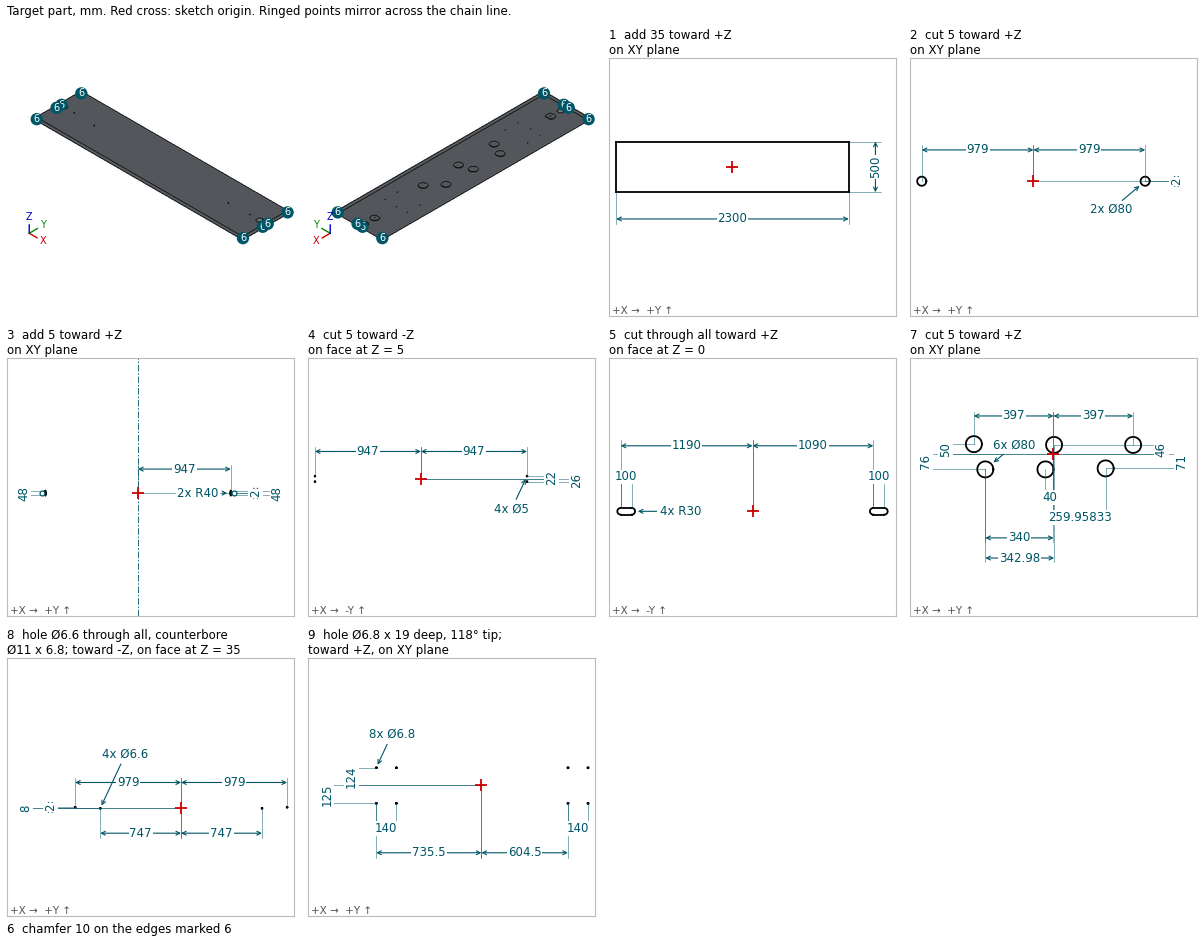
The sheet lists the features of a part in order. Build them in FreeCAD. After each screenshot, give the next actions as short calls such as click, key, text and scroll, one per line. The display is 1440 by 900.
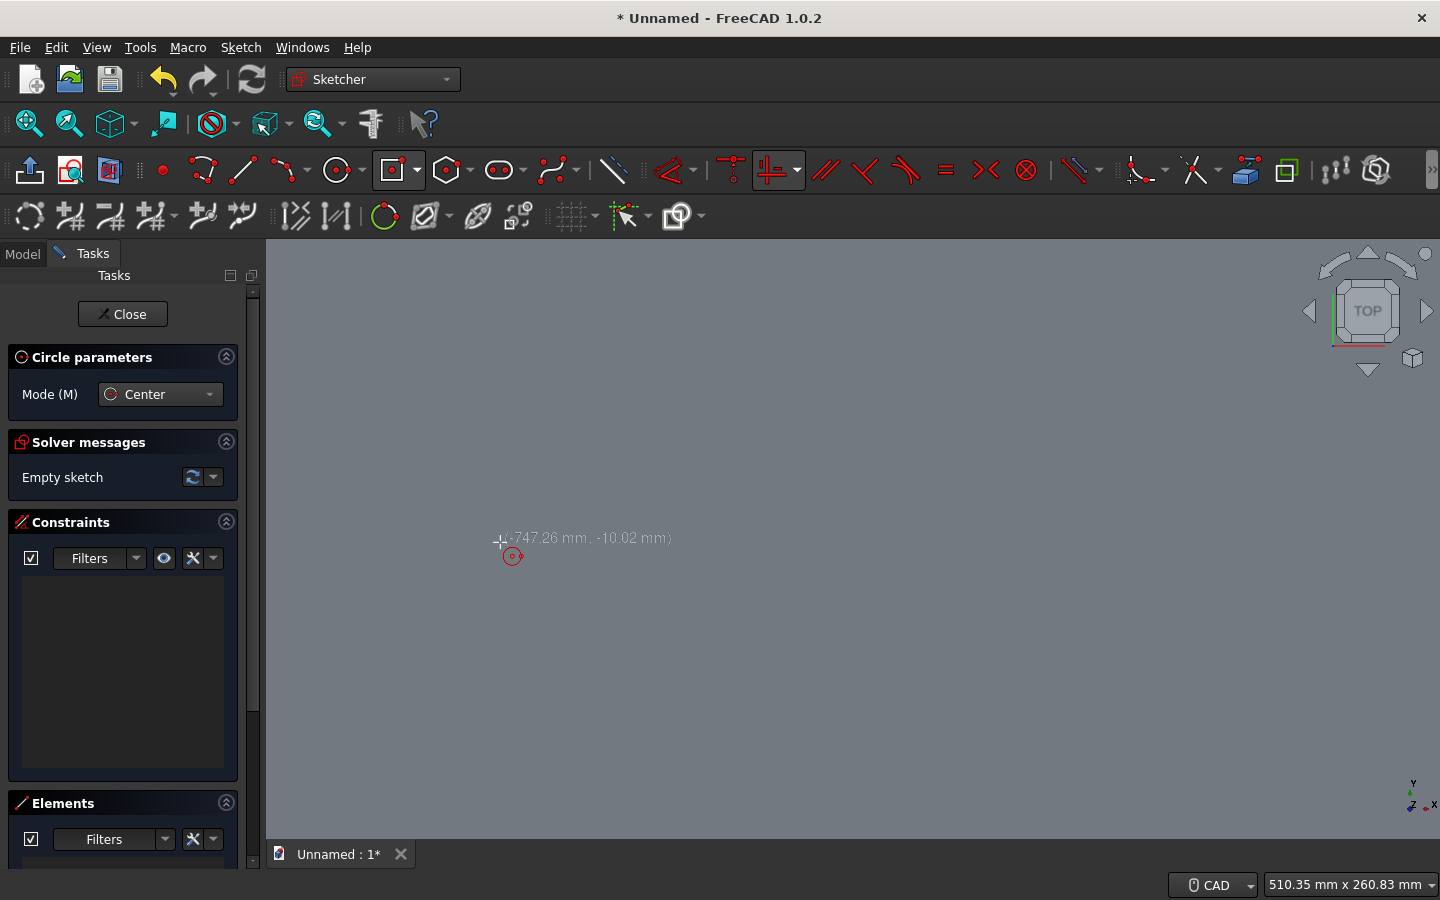
click(501, 538)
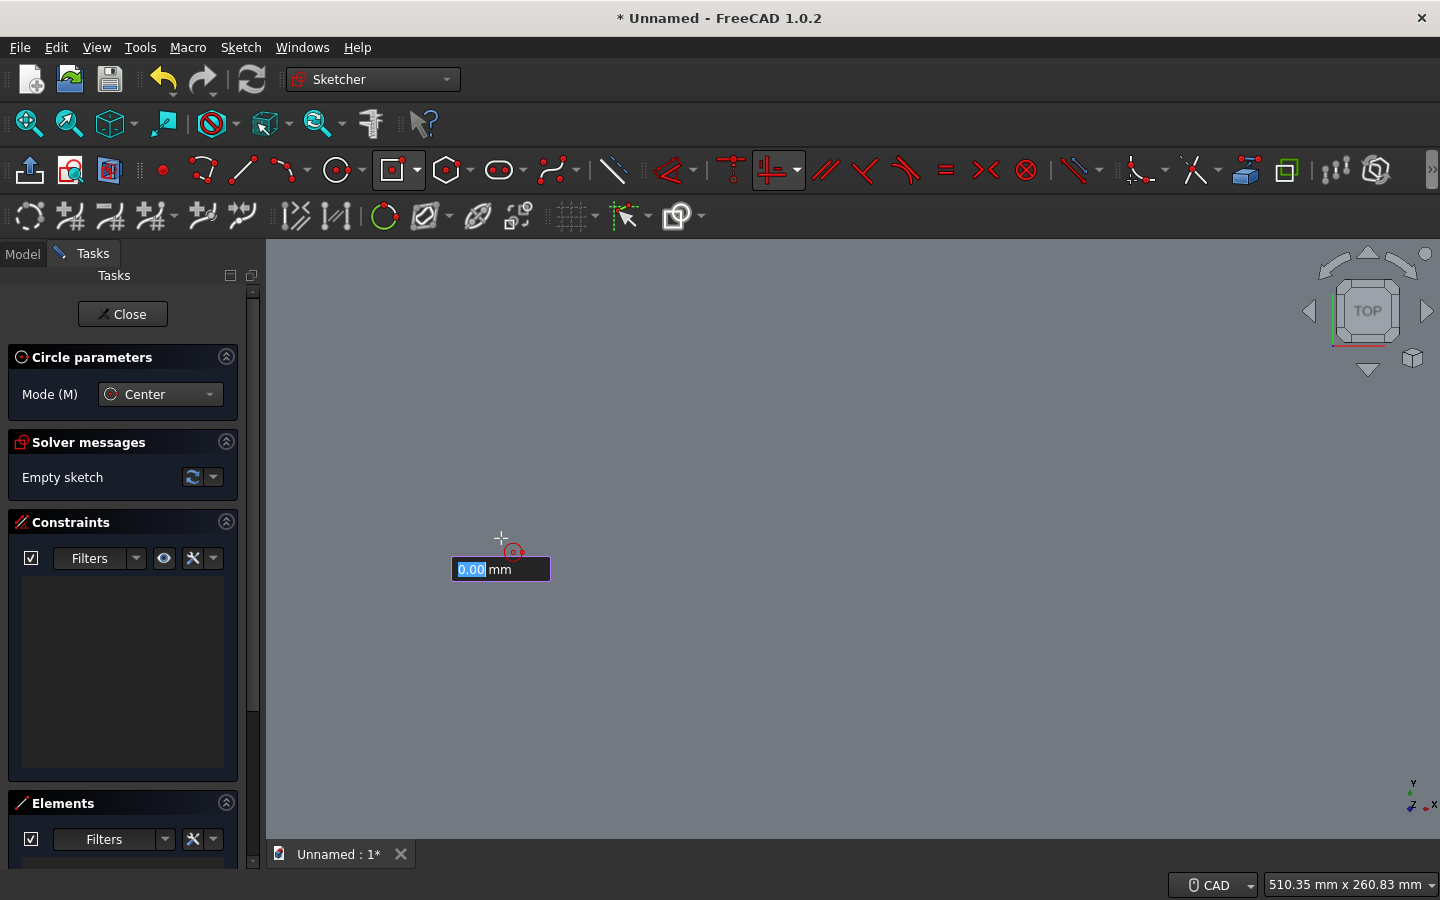
scroll(506, 543, up, 4)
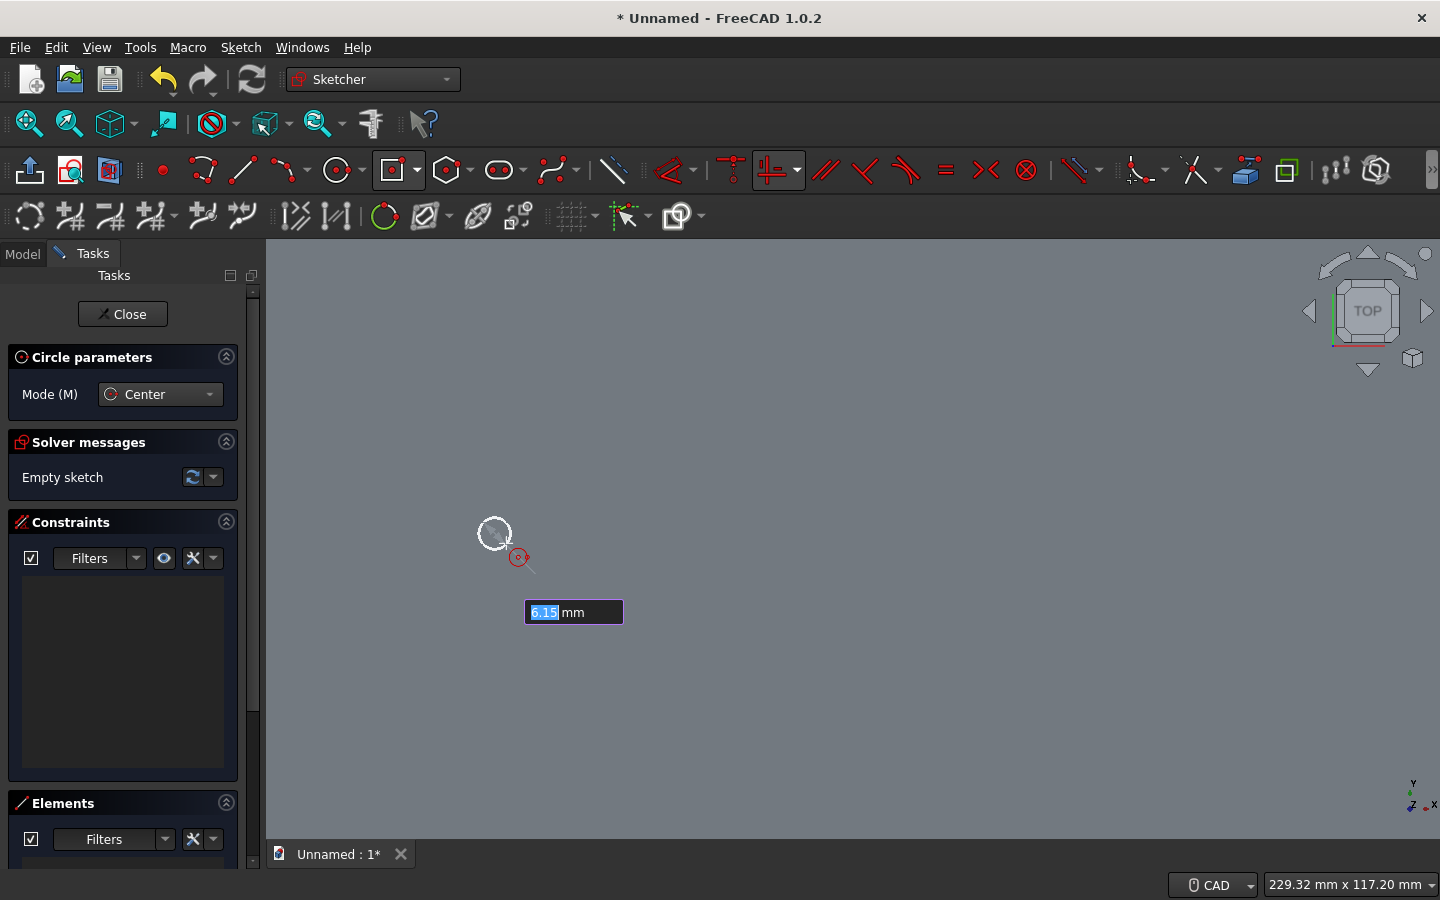
click(506, 543)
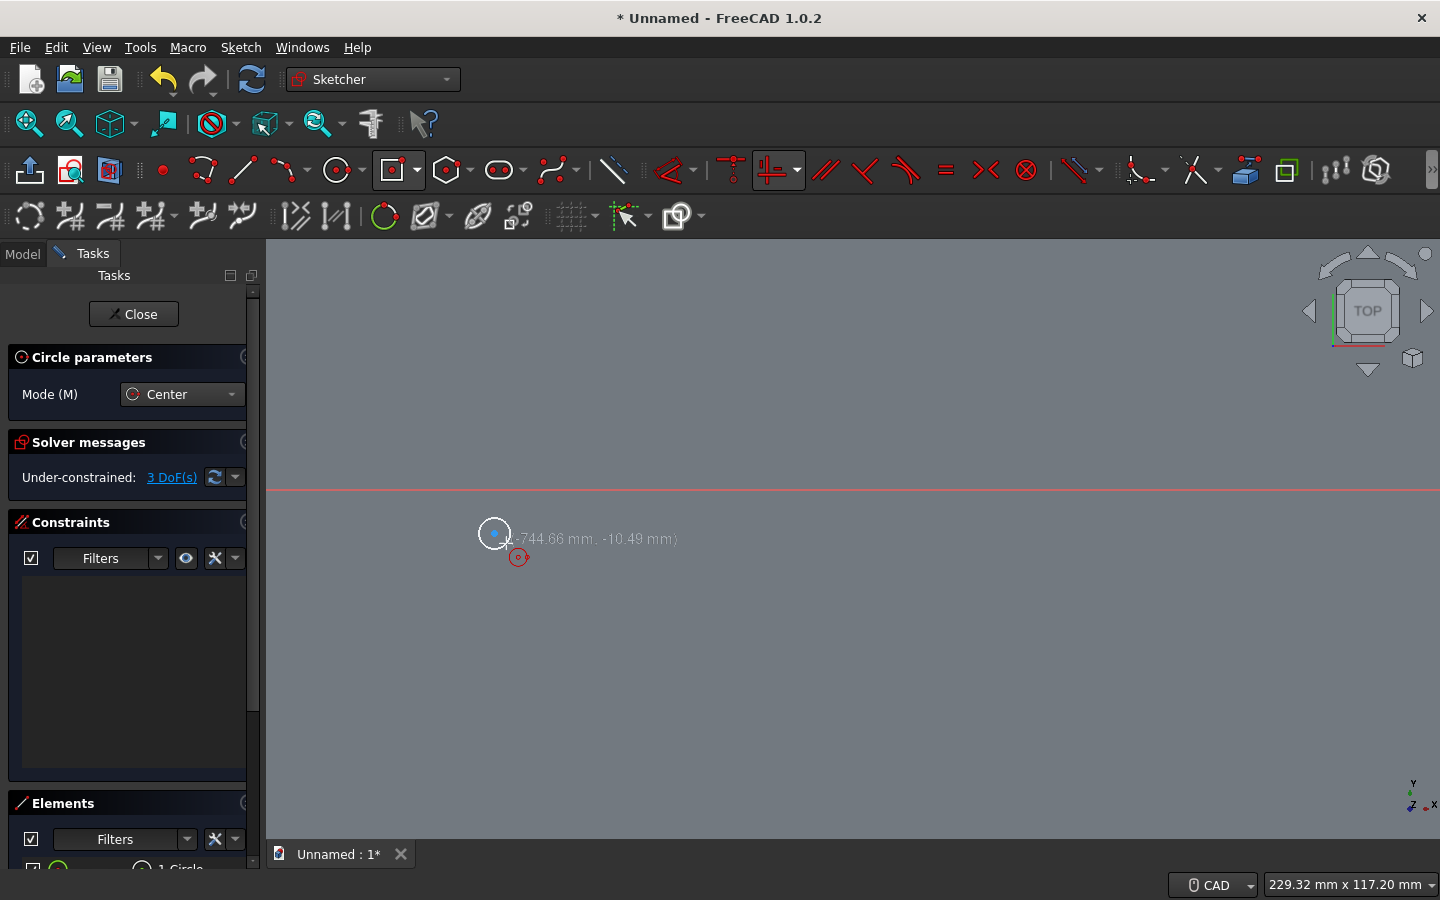
scroll(501, 542, down, 13)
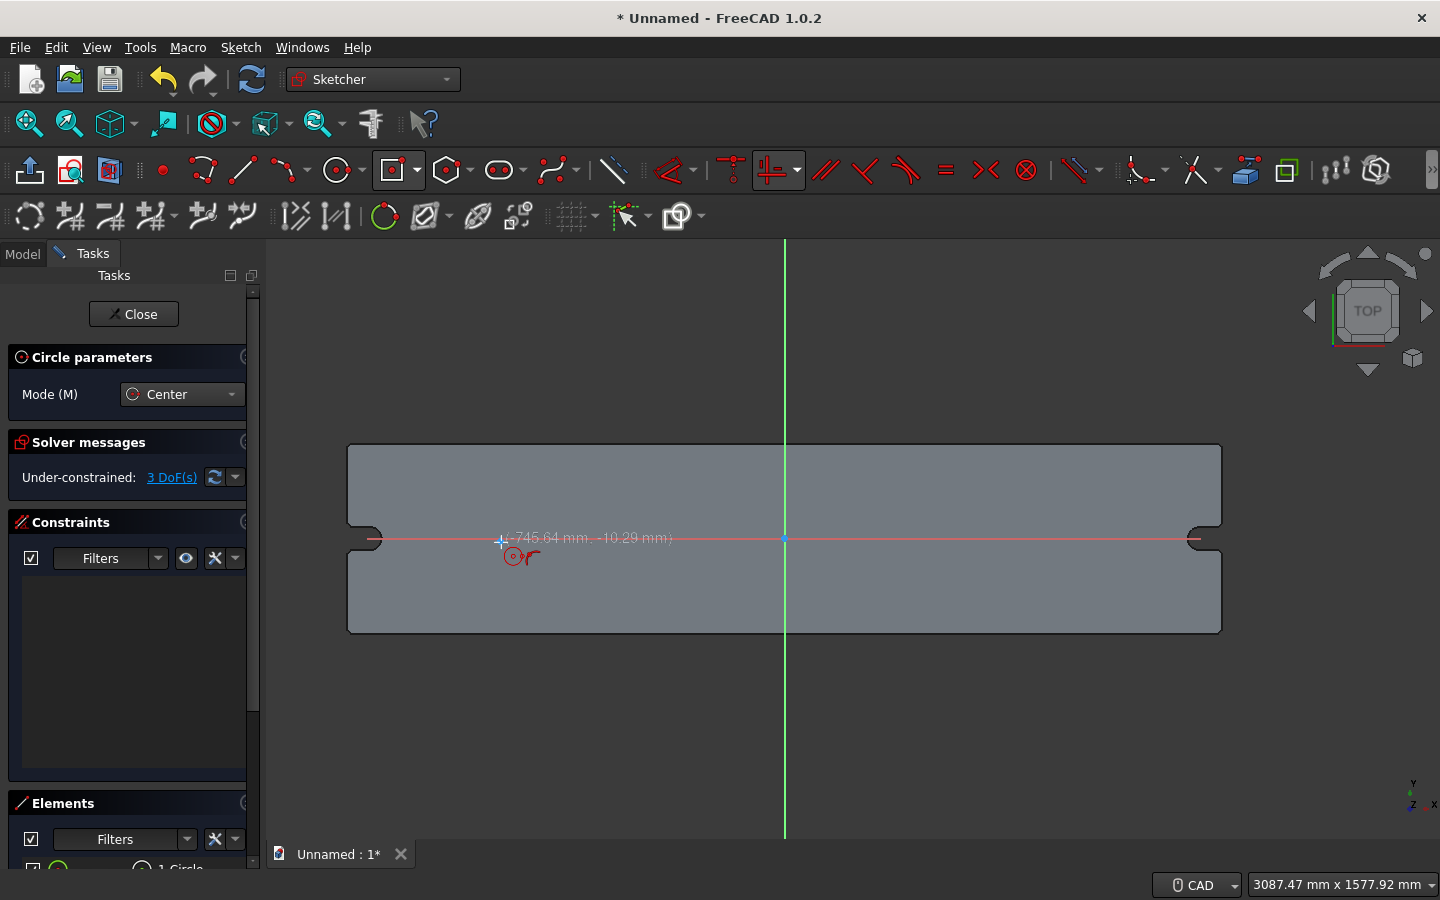
scroll(1069, 542, up, 15)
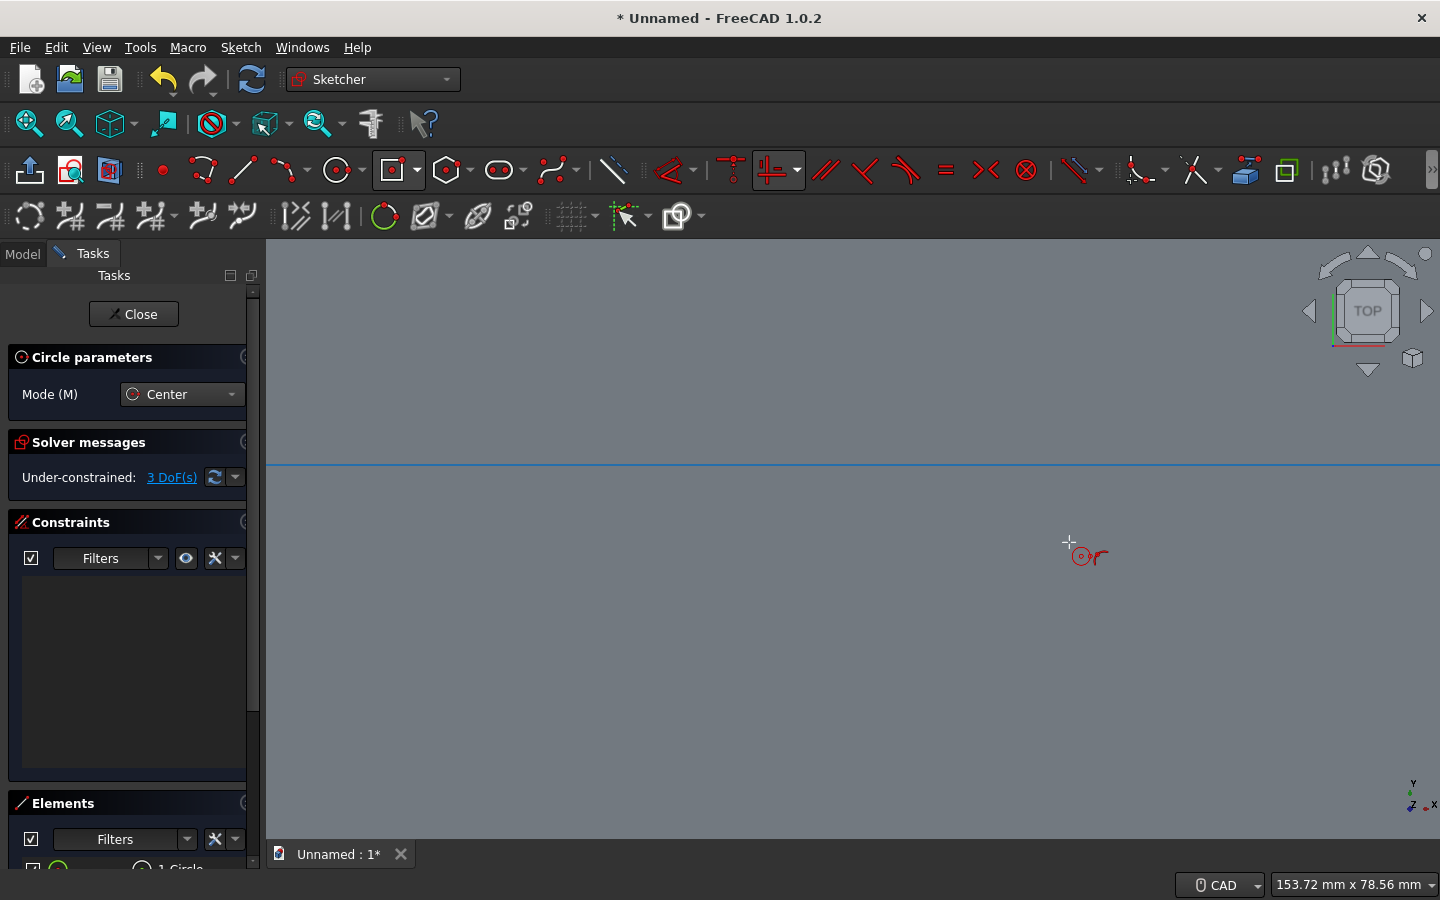
scroll(1069, 542, down, 15)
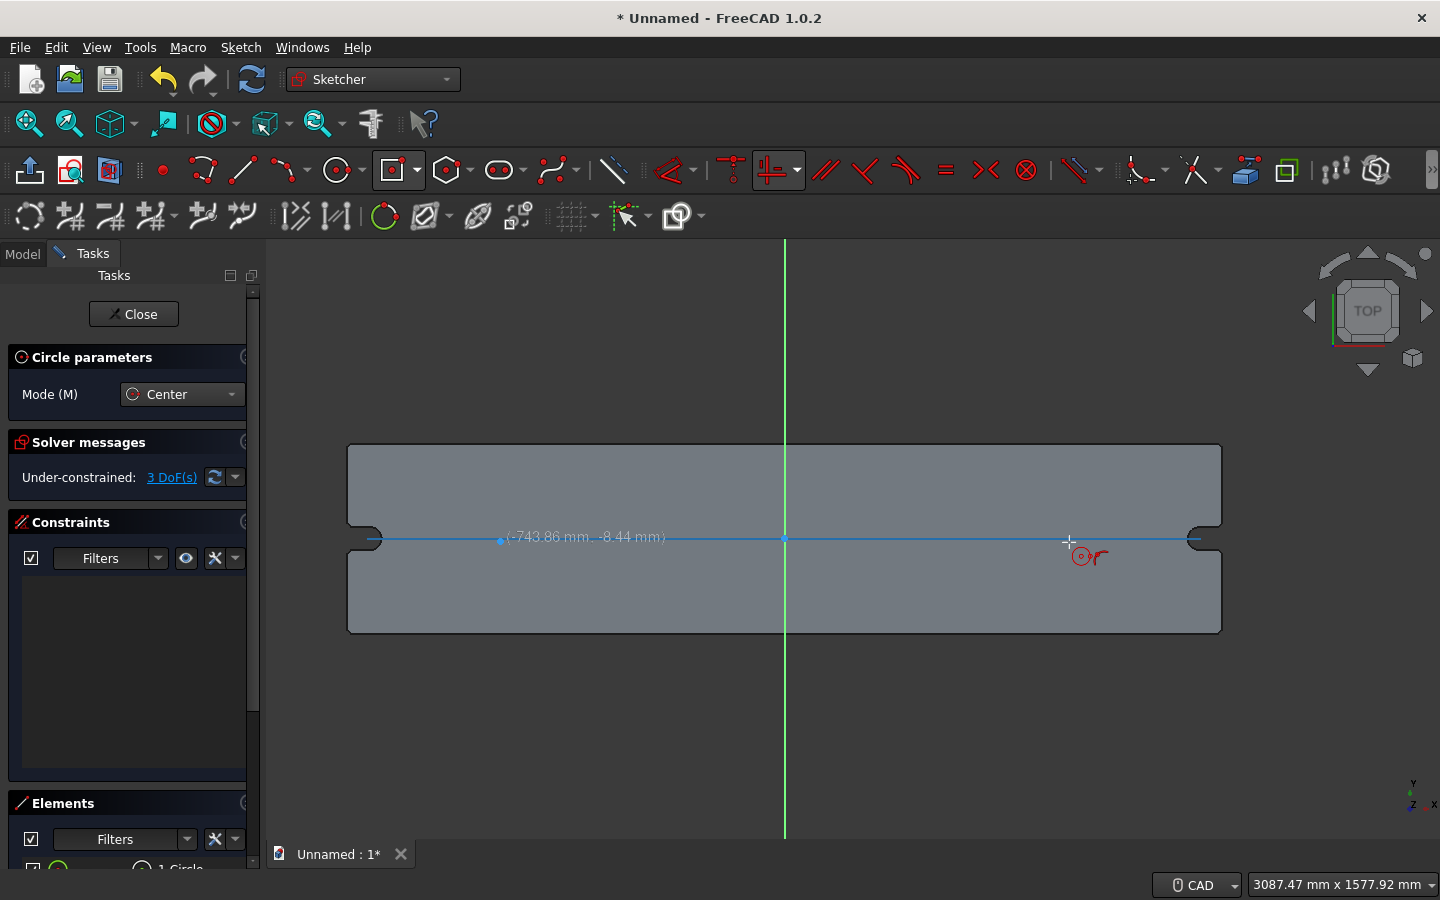
scroll(1069, 542, up, 9)